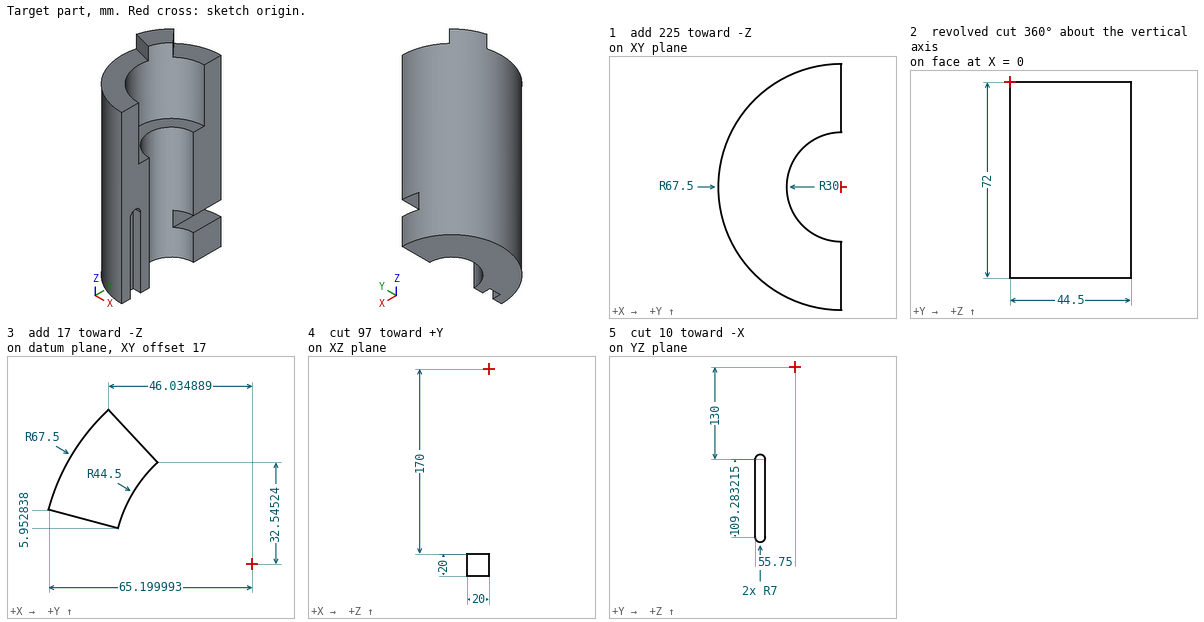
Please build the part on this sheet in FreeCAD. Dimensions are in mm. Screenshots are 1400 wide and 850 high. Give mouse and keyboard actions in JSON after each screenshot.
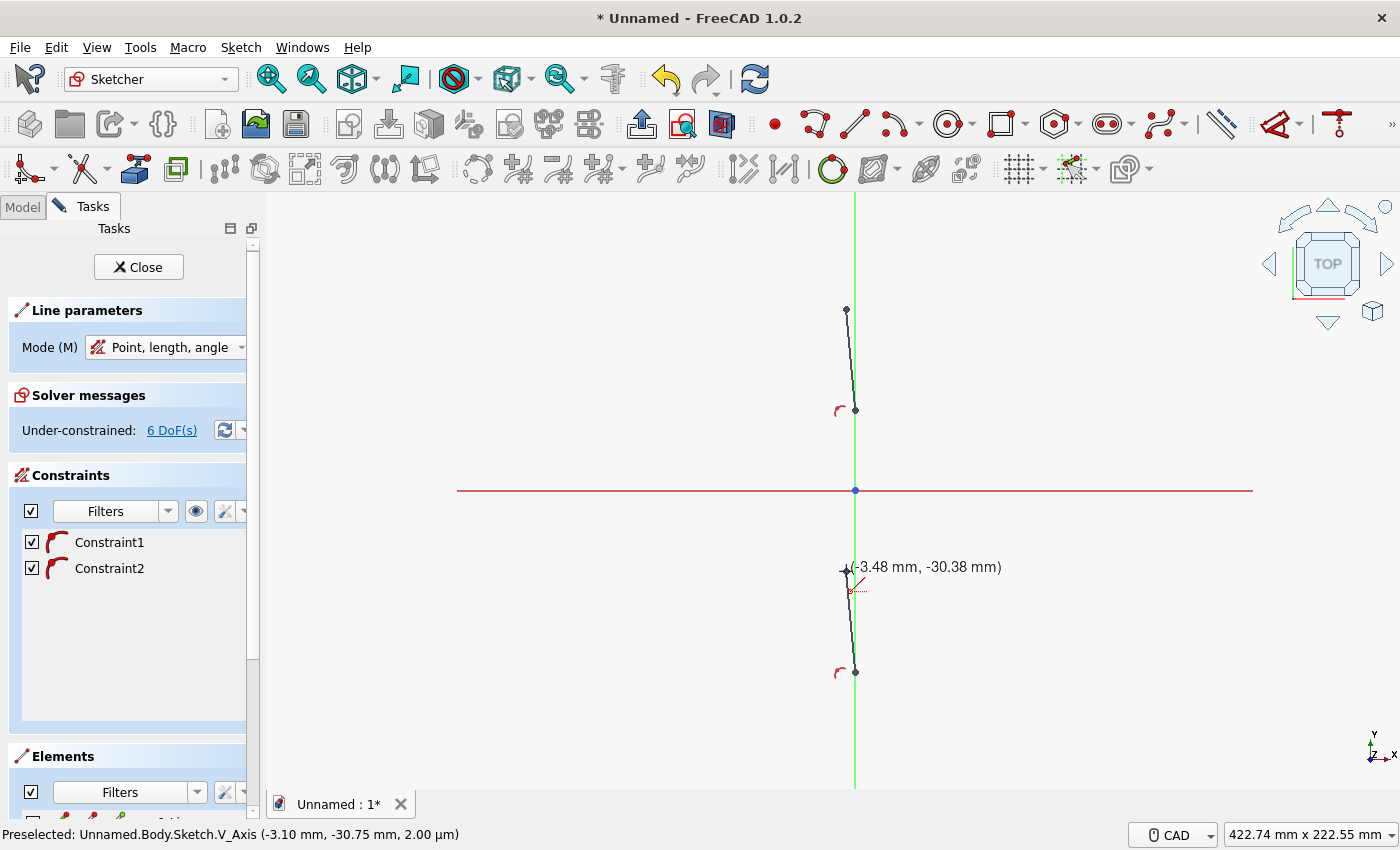
{"action": "key", "text": "g 3 a"}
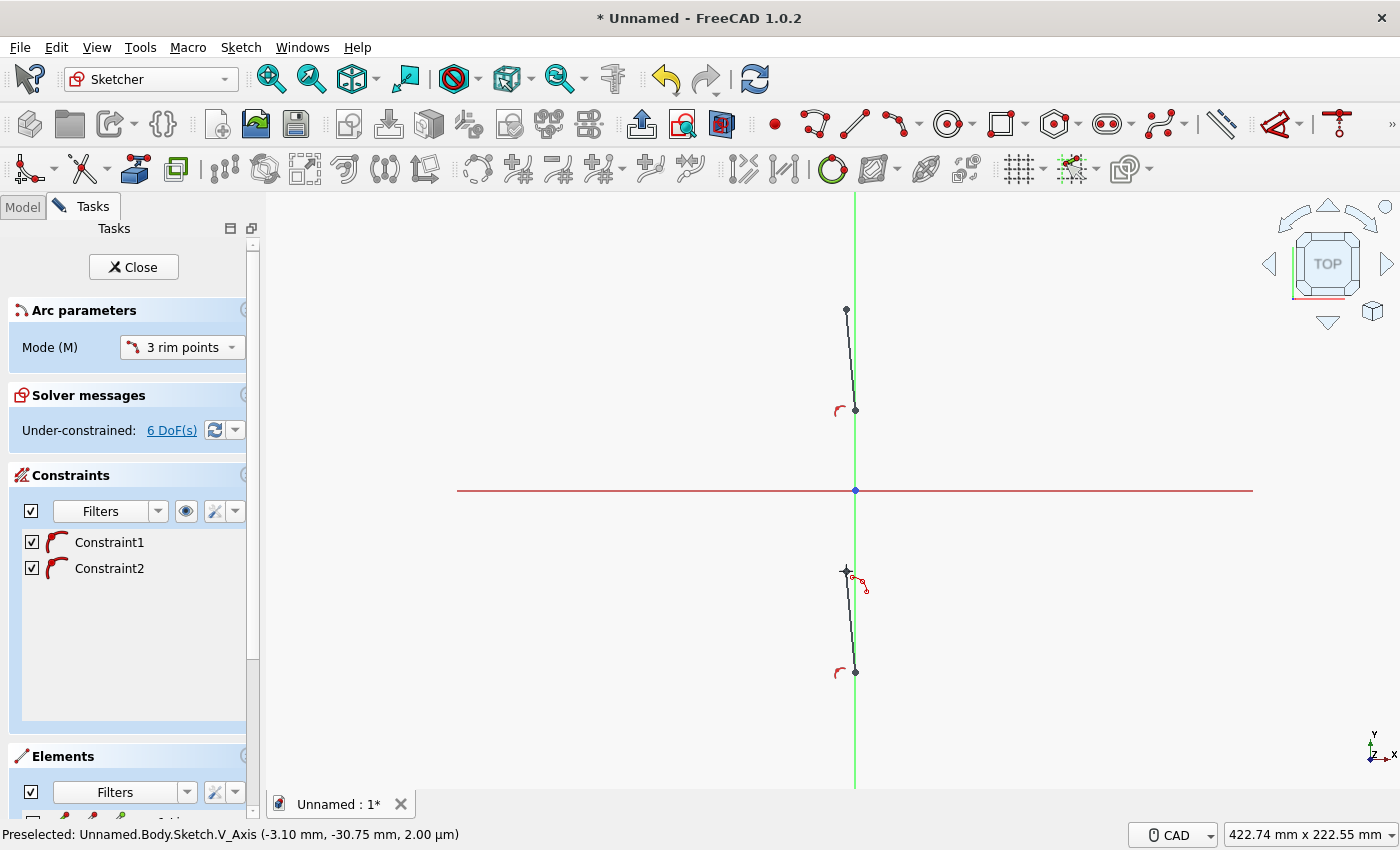
{"action": "left_click", "coordinate": [846, 310]}
{"action": "left_click", "coordinate": [855, 673]}
{"action": "left_click", "coordinate": [683, 435]}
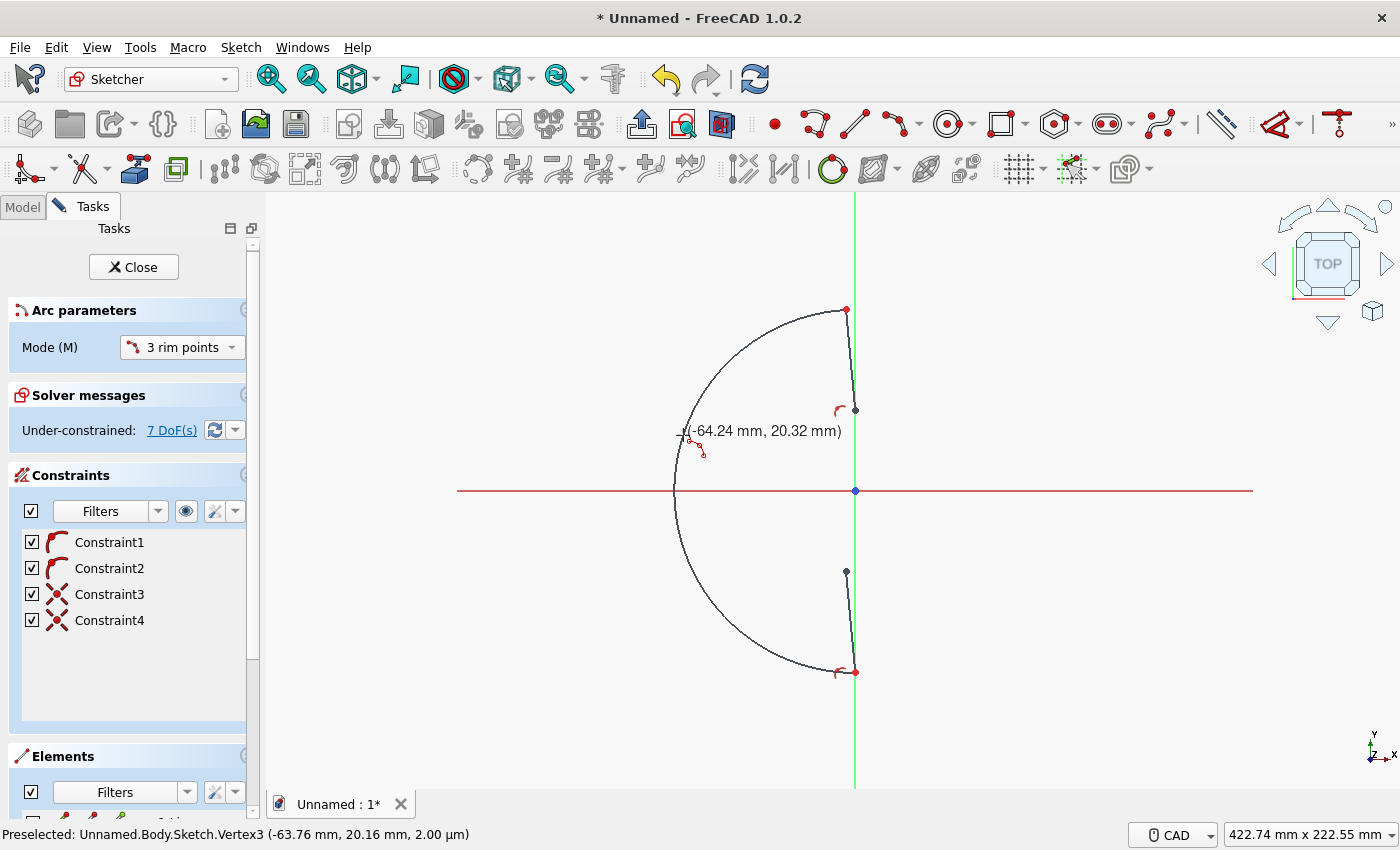
{"action": "left_click", "coordinate": [846, 572]}
{"action": "left_click", "coordinate": [855, 411]}
{"action": "left_click", "coordinate": [779, 466]}
{"action": "key", "text": "Escape"}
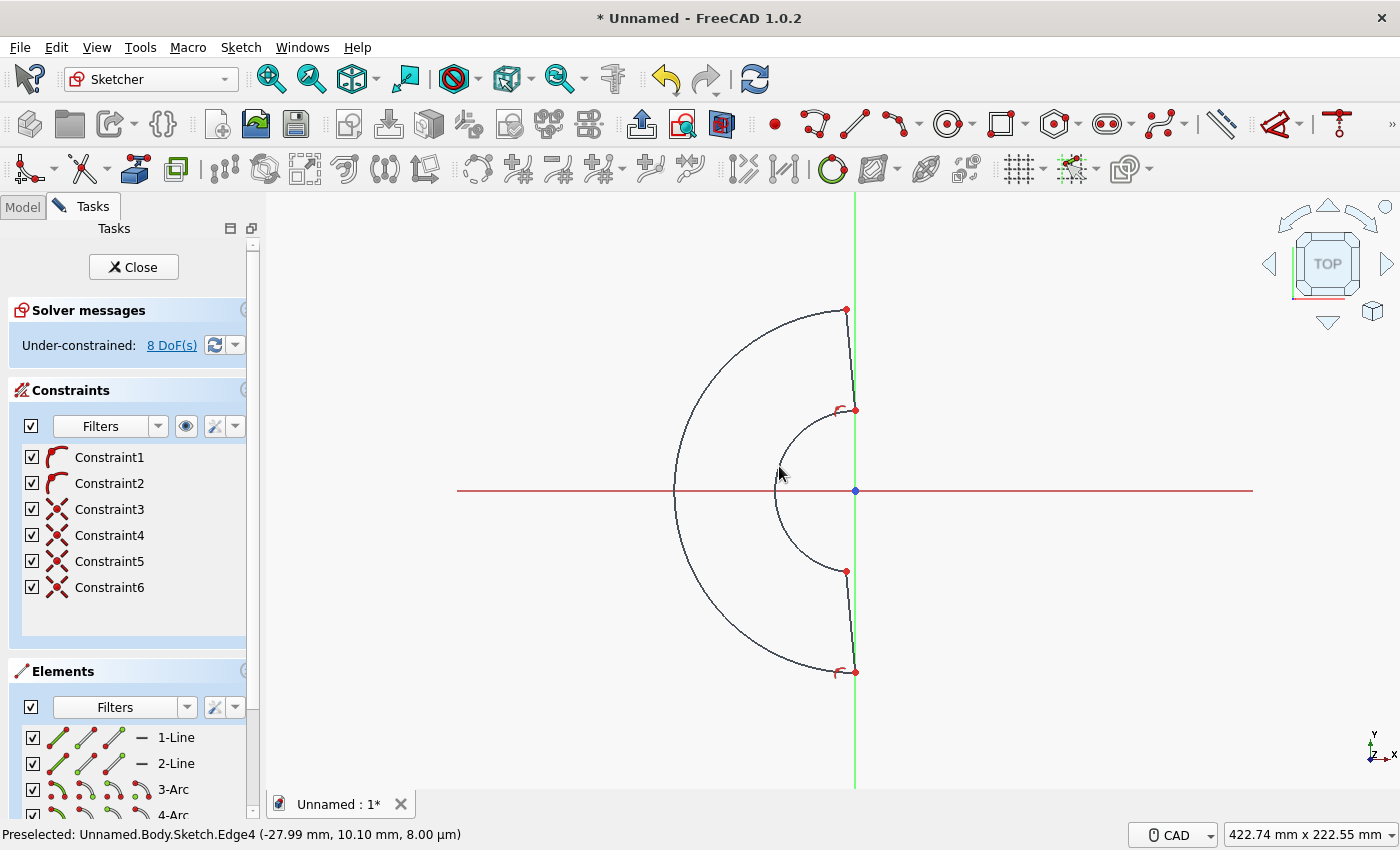
{"action": "left_click", "coordinate": [853, 381]}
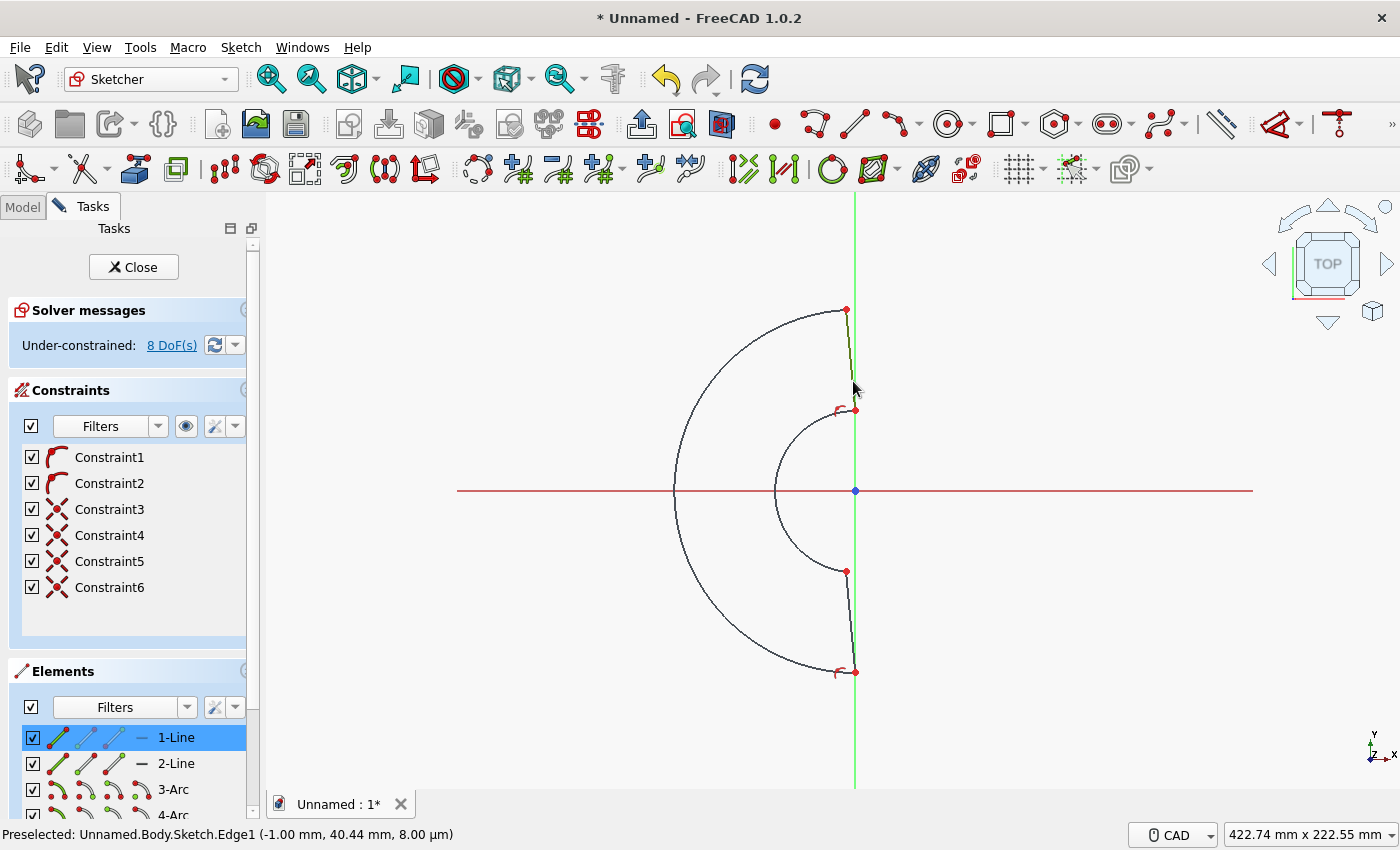
{"action": "key", "text": "v"}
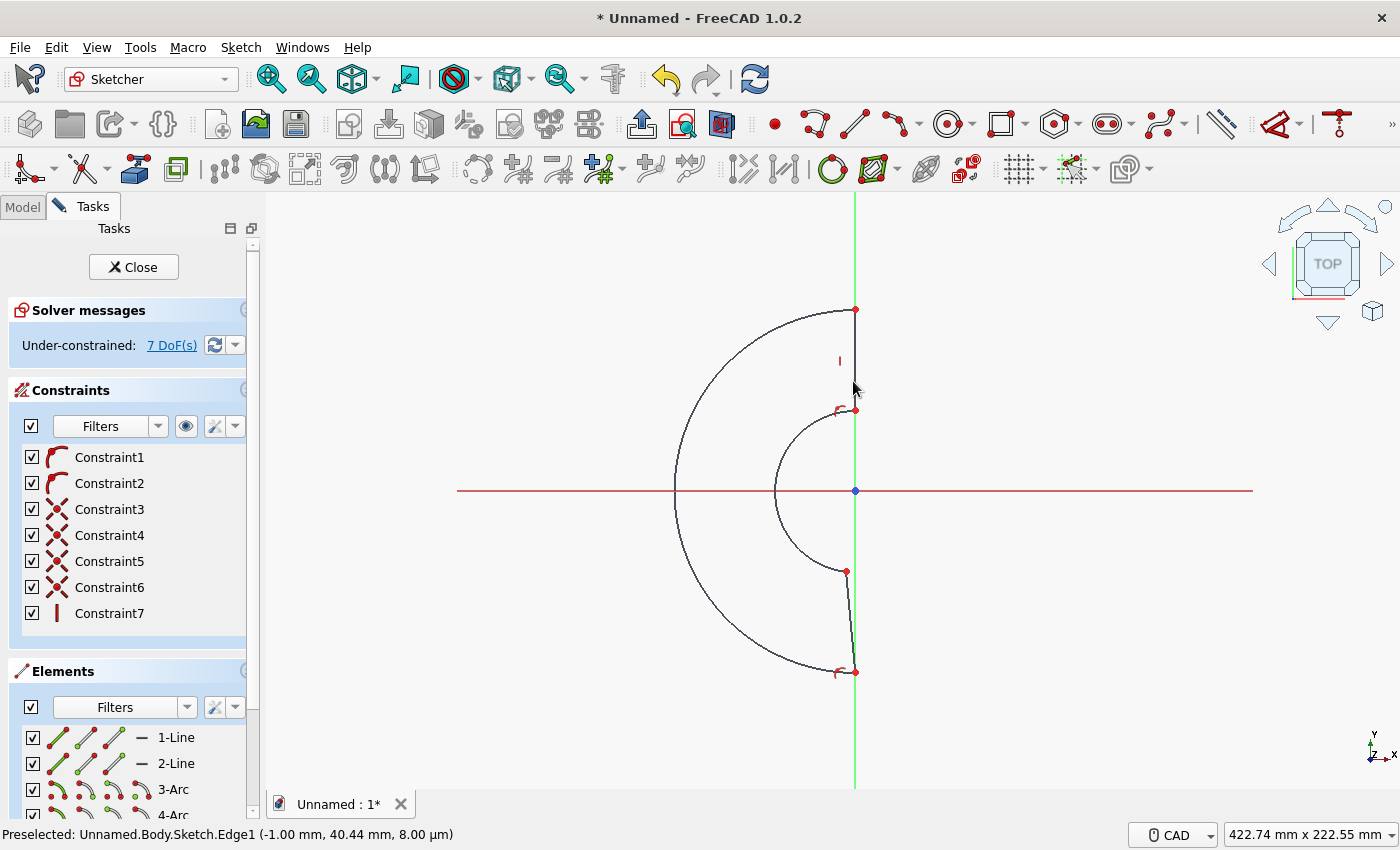
{"action": "left_click", "coordinate": [853, 643]}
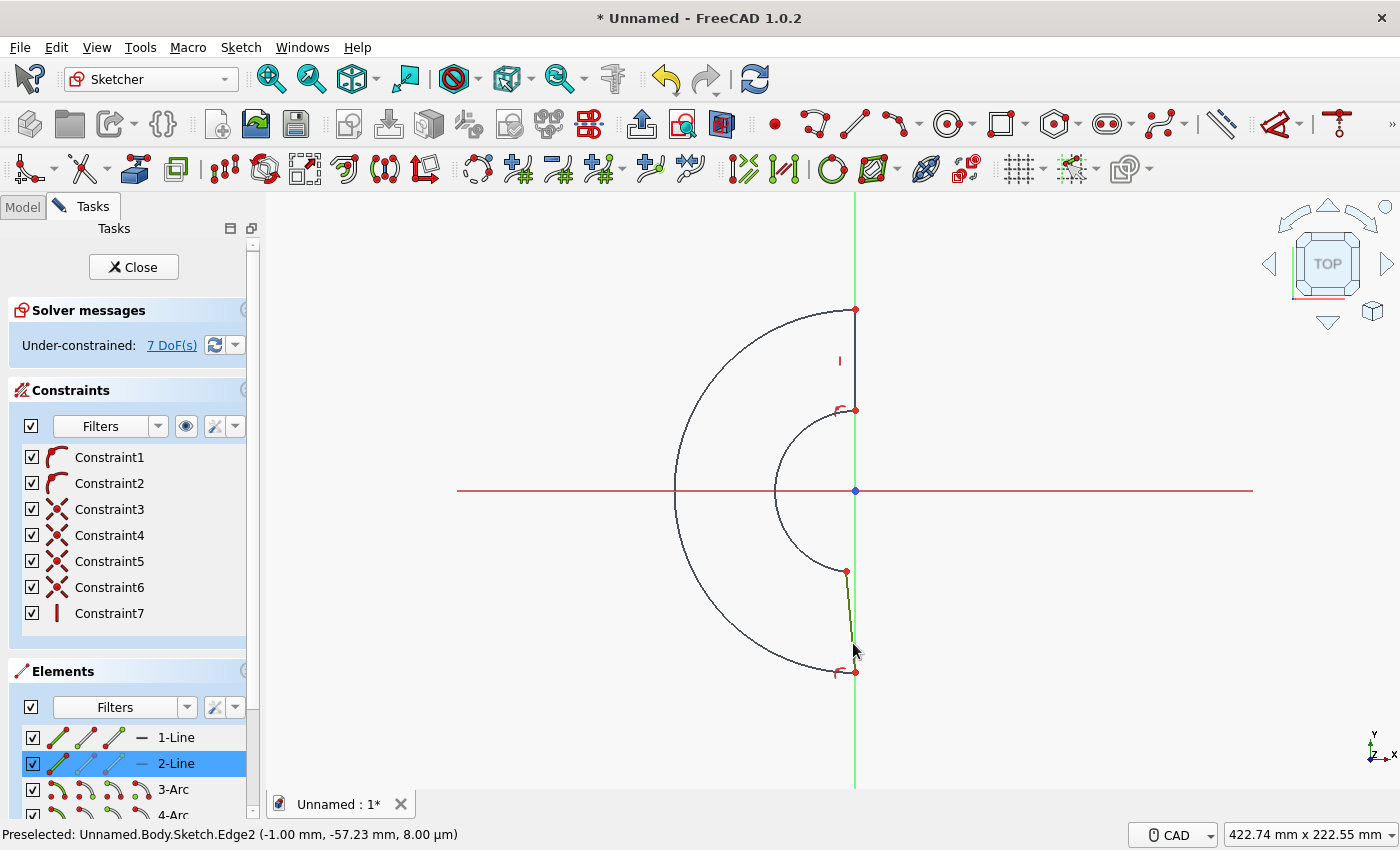
{"action": "key", "text": "v"}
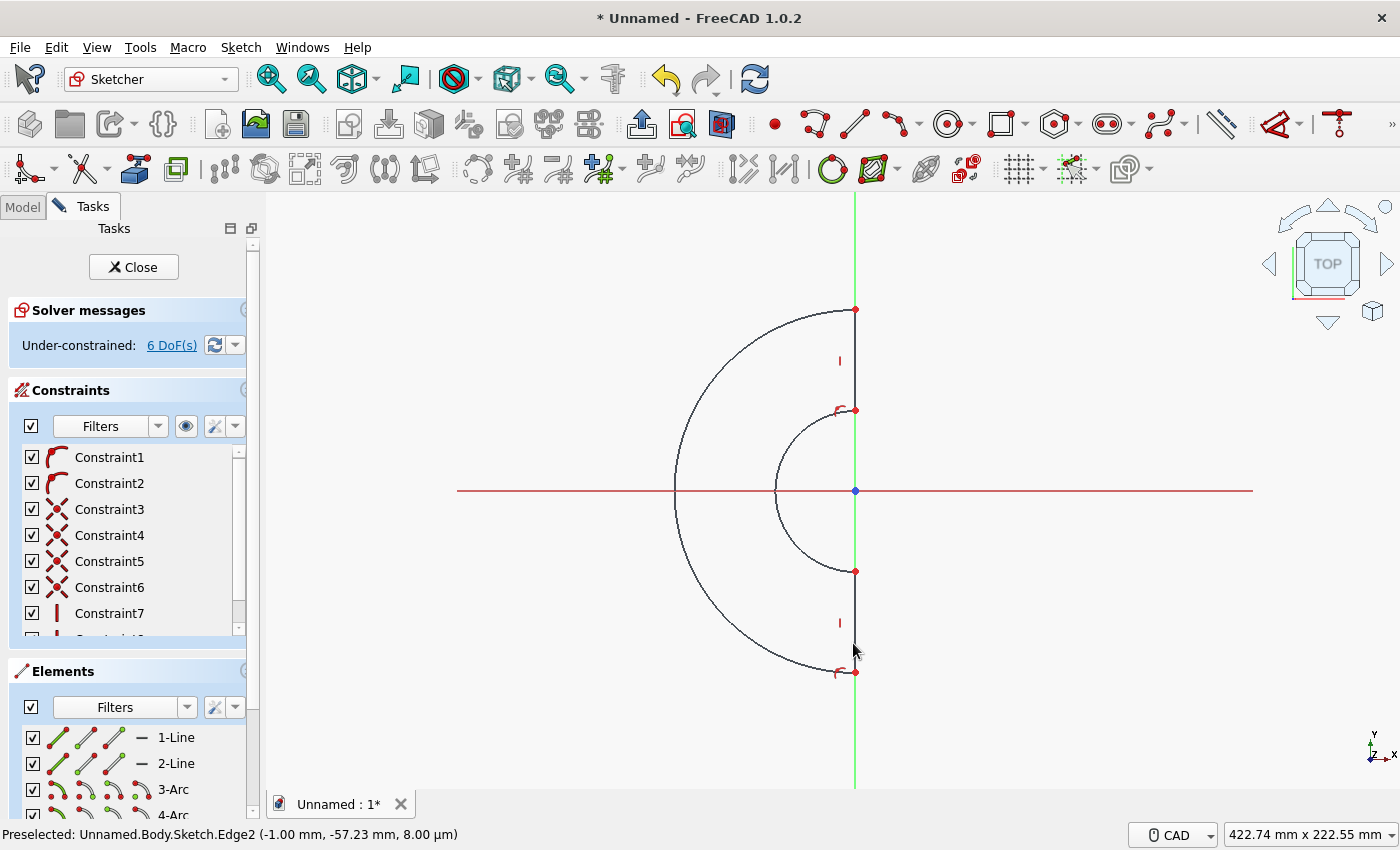
{"action": "left_click", "coordinate": [709, 385]}